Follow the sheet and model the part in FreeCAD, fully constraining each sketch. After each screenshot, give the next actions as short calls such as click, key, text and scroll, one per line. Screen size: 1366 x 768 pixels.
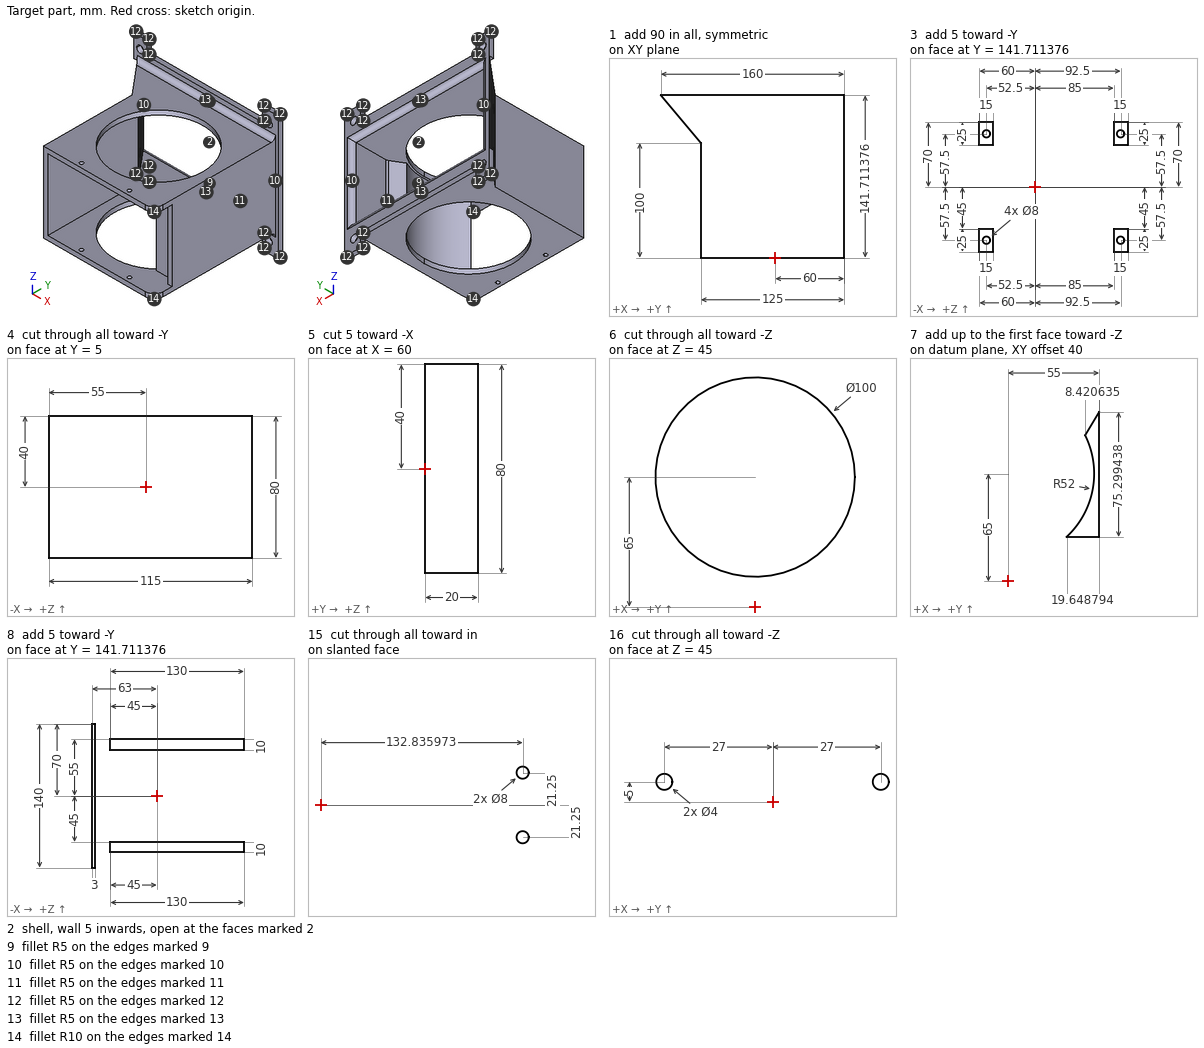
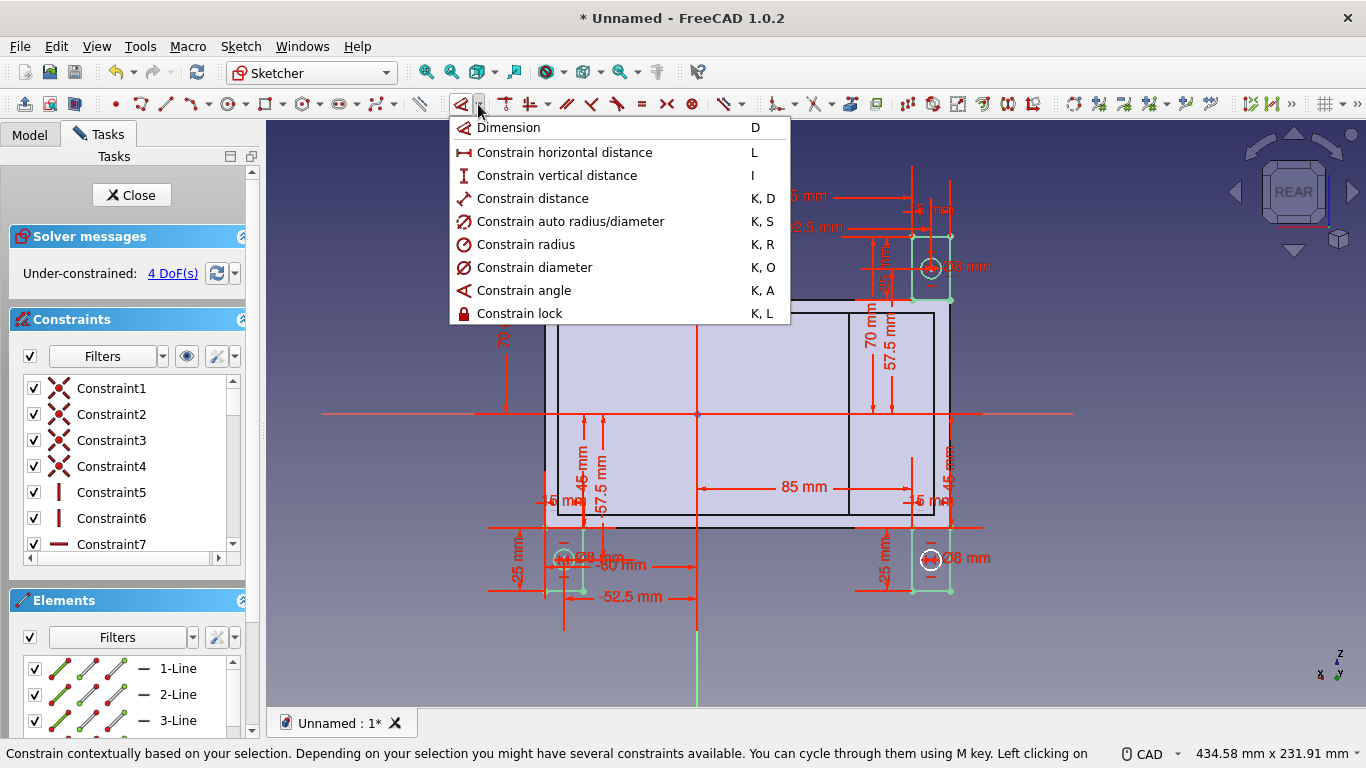
click(620, 152)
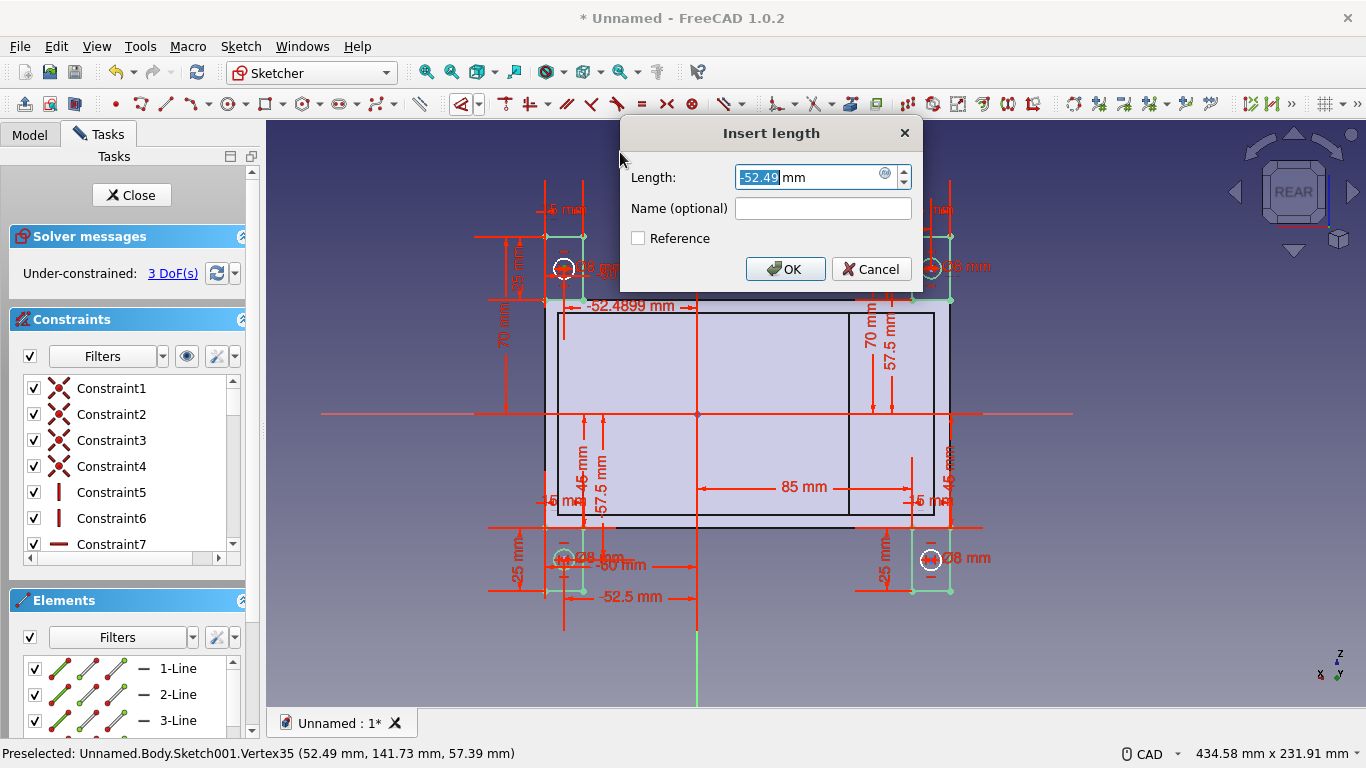
text(-52.5)
key(Return)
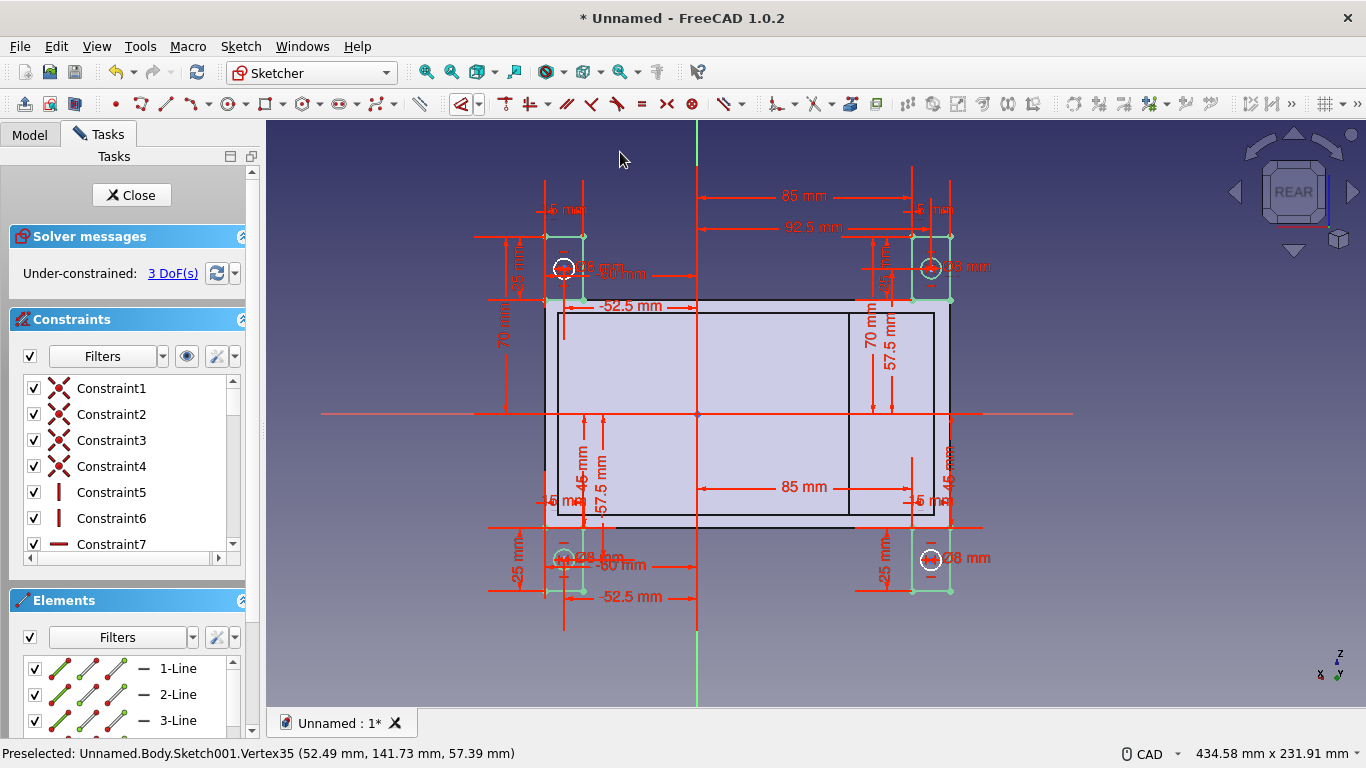
click(564, 269)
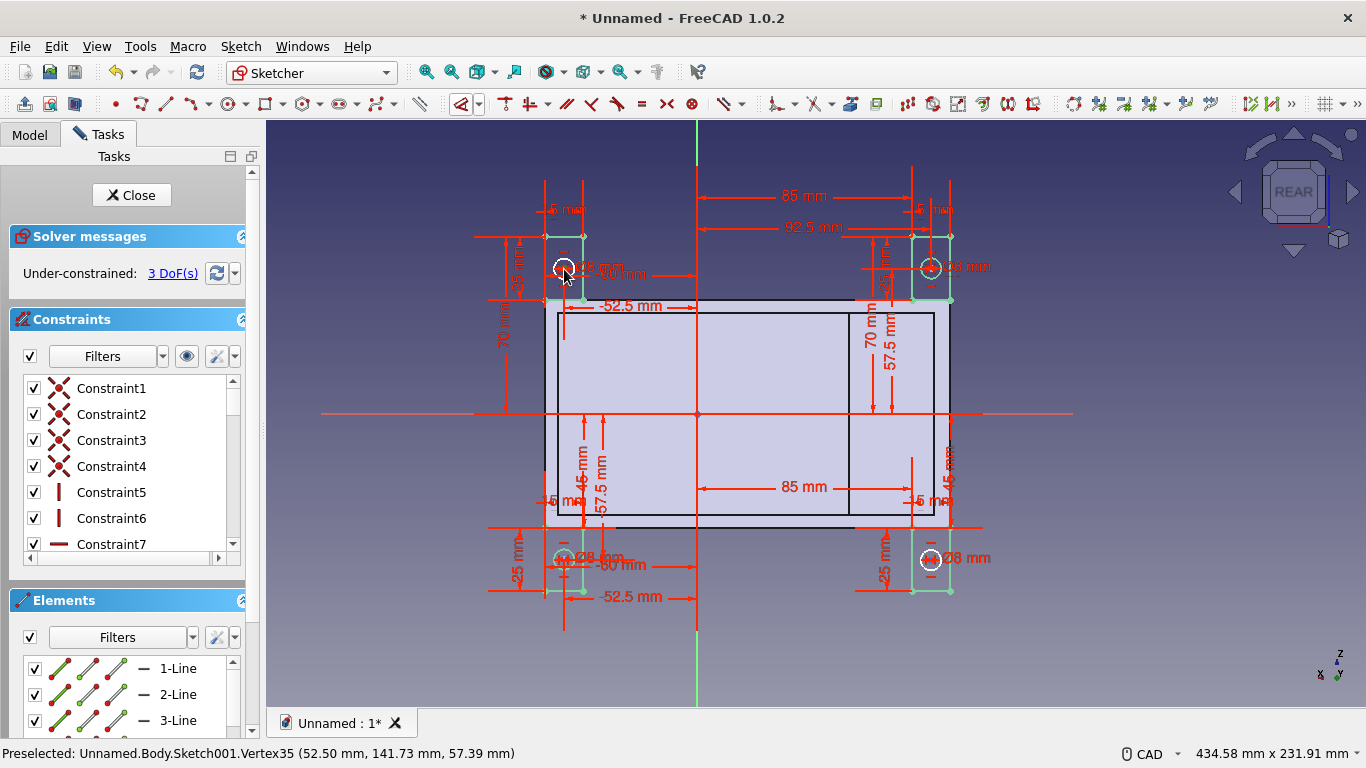
key(i)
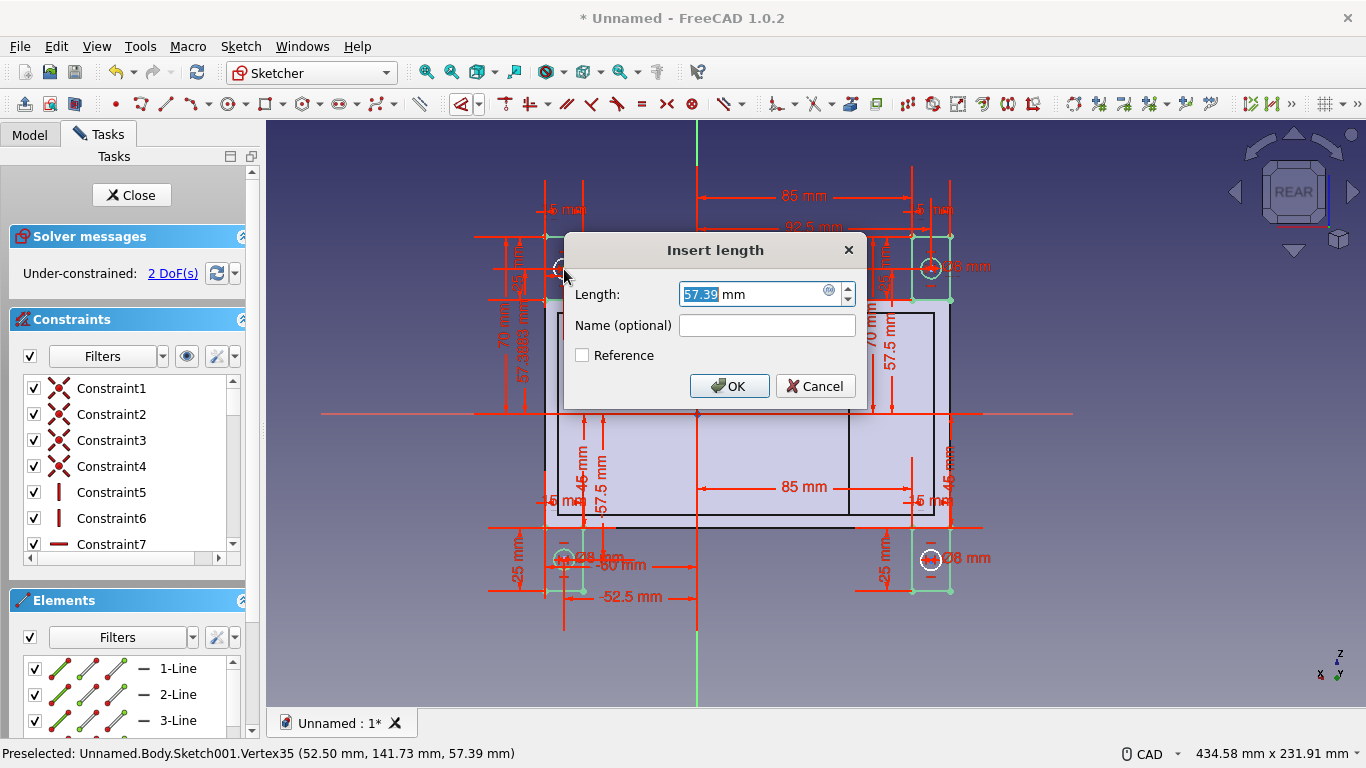
text(57.5)
key(Return)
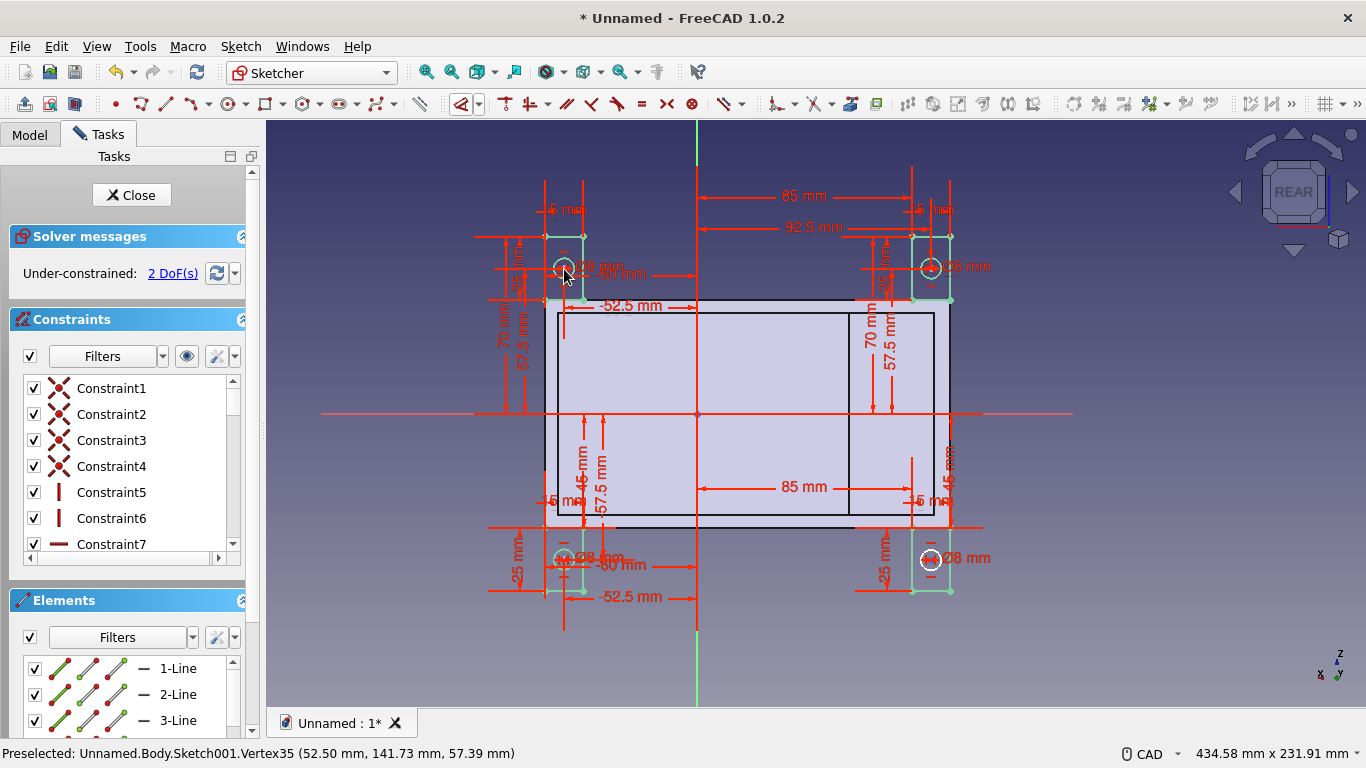
click(931, 560)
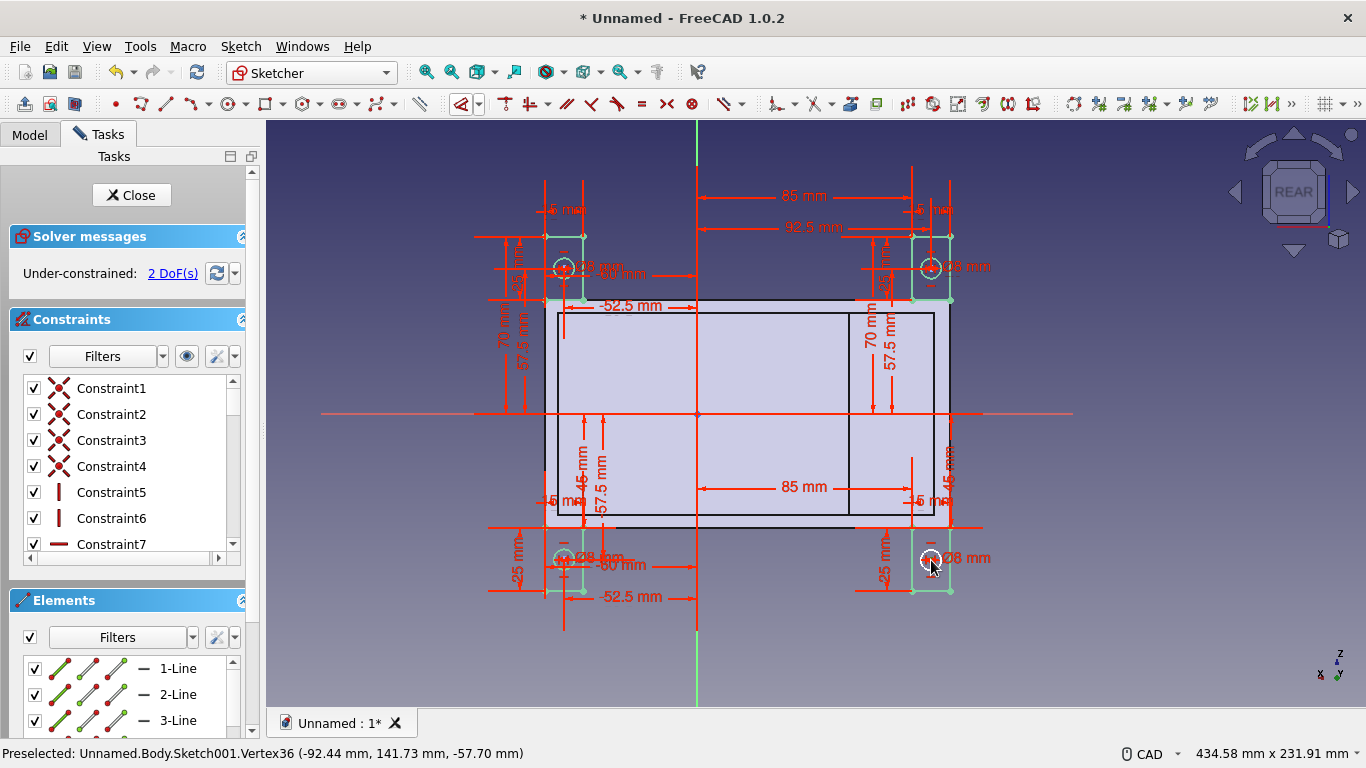
key(l)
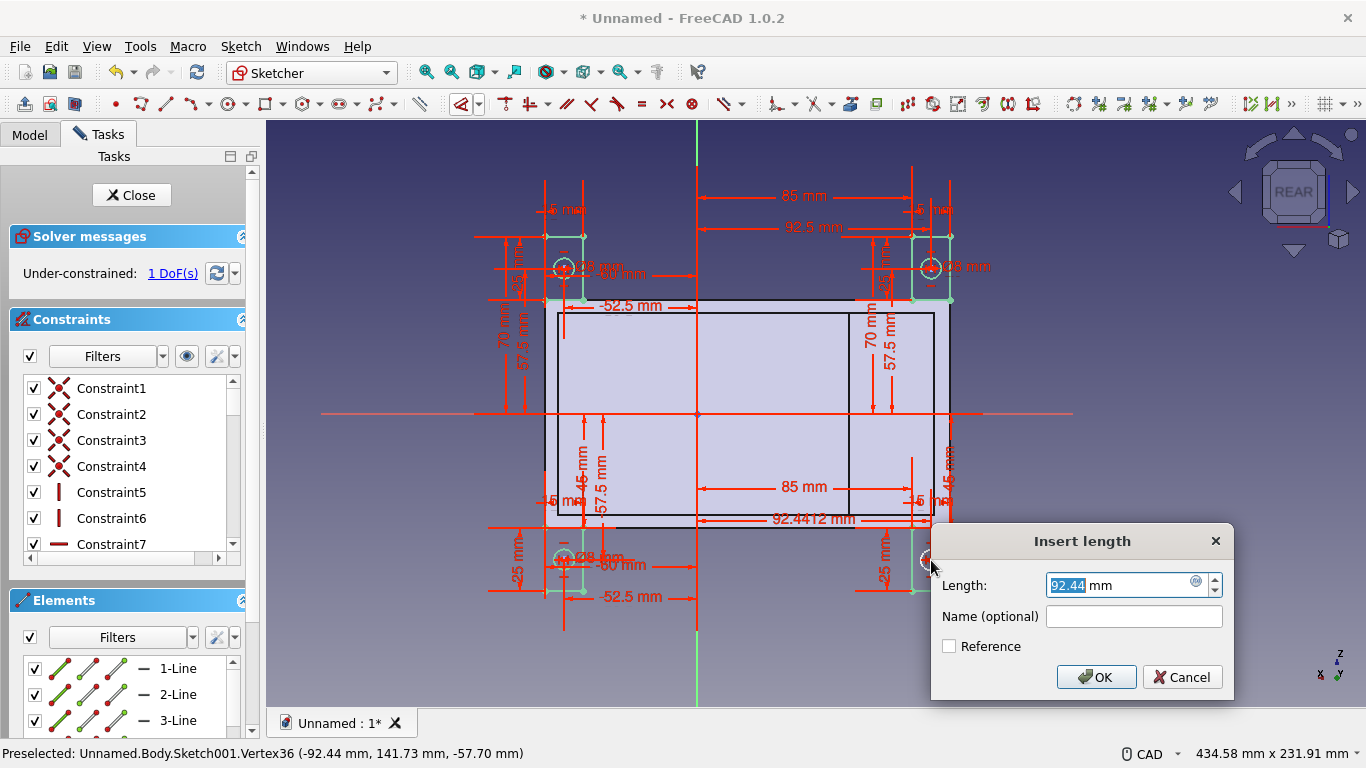
text(92.5)
key(Return)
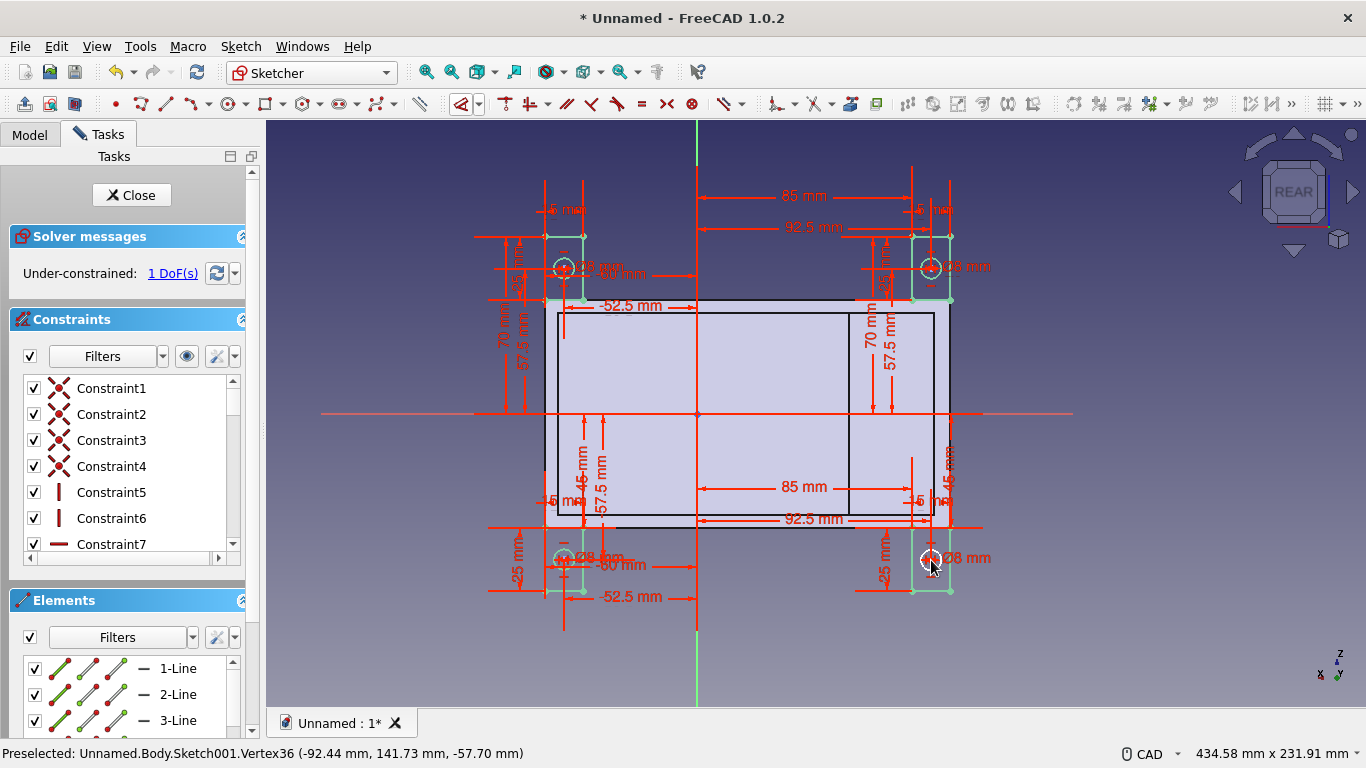
click(931, 560)